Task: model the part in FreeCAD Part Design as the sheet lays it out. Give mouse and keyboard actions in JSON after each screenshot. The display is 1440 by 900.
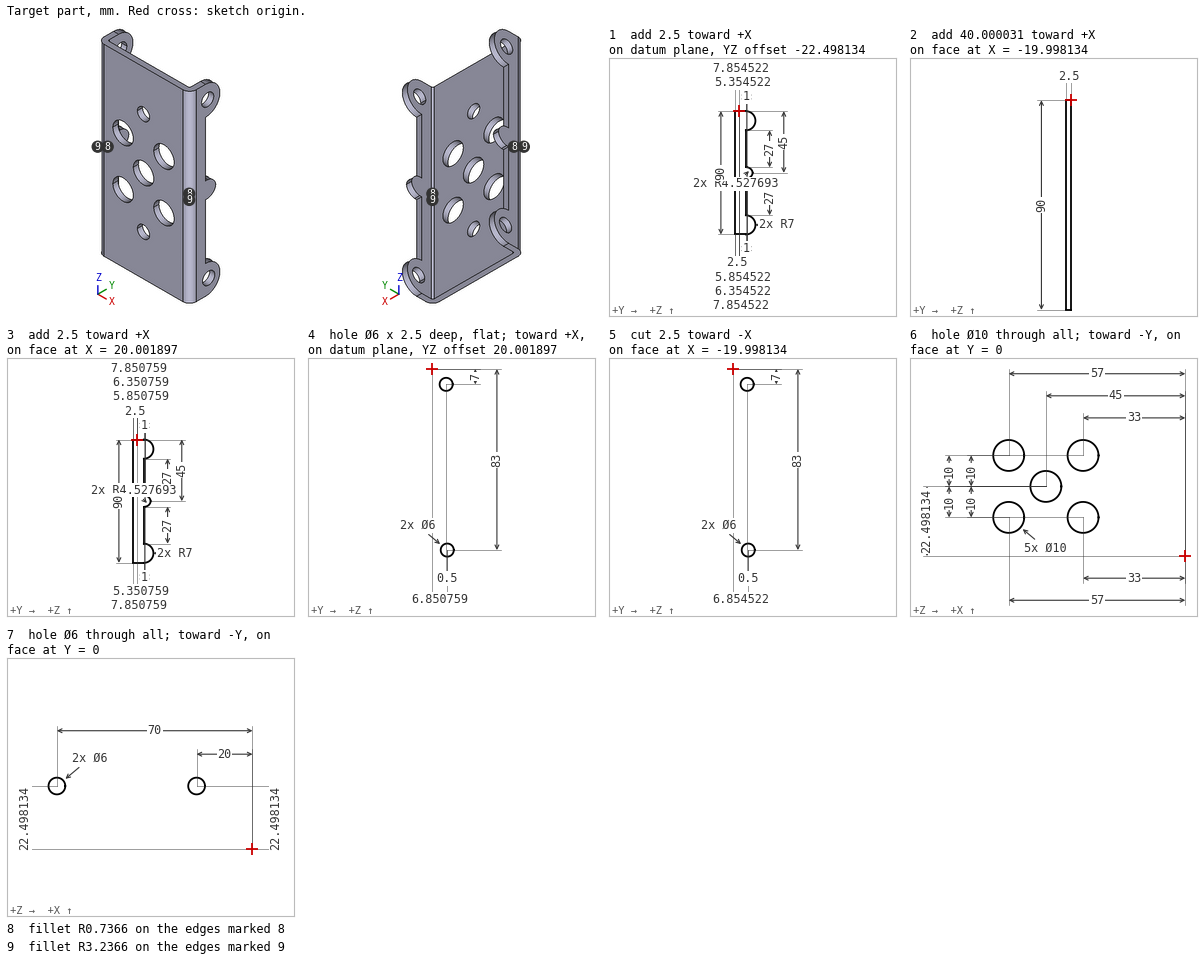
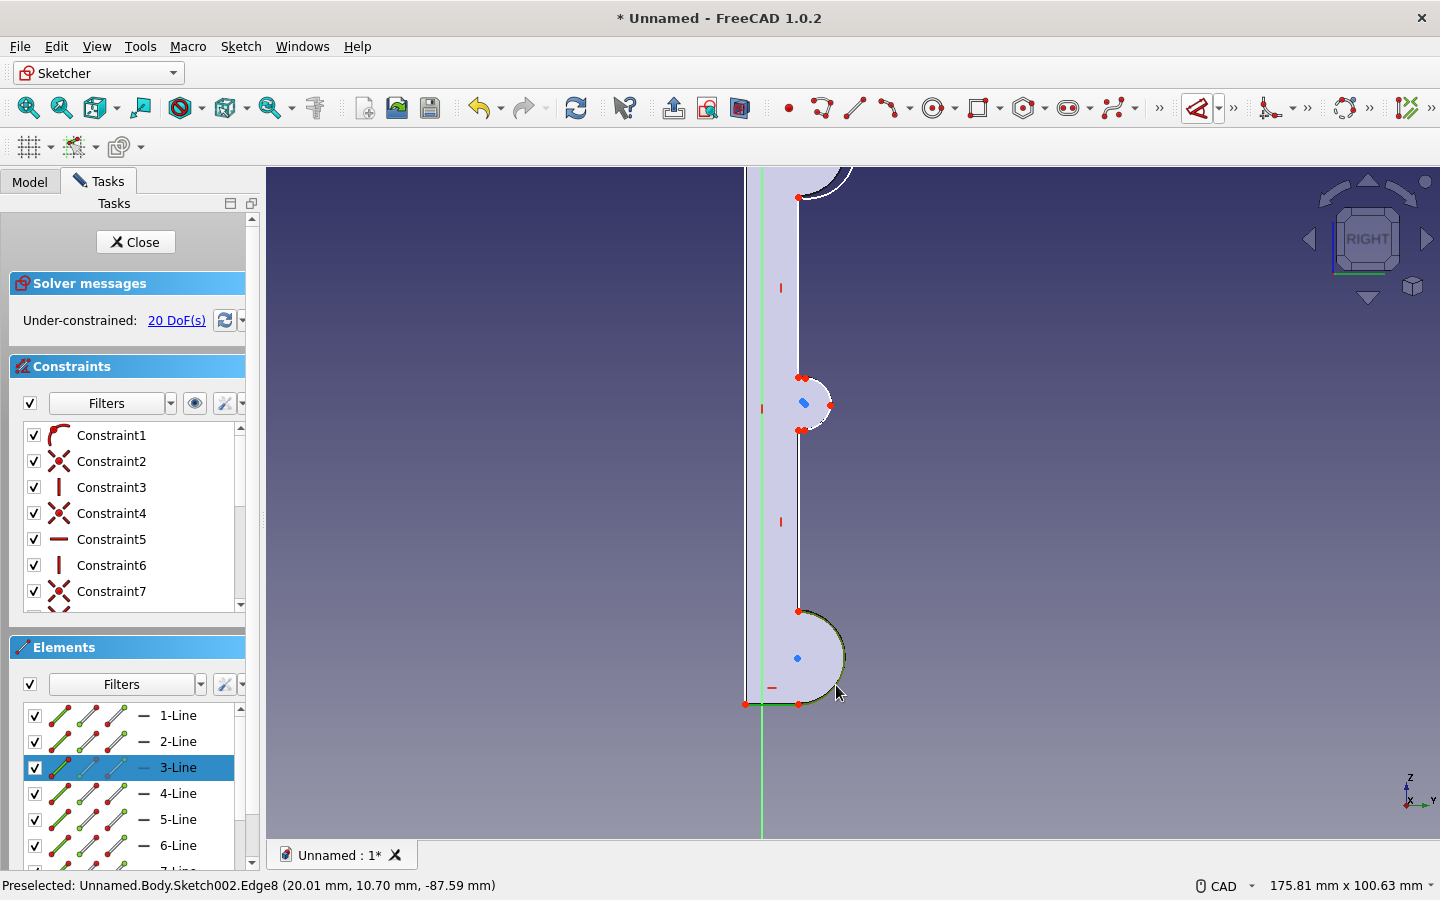
{"action": "key", "text": "t"}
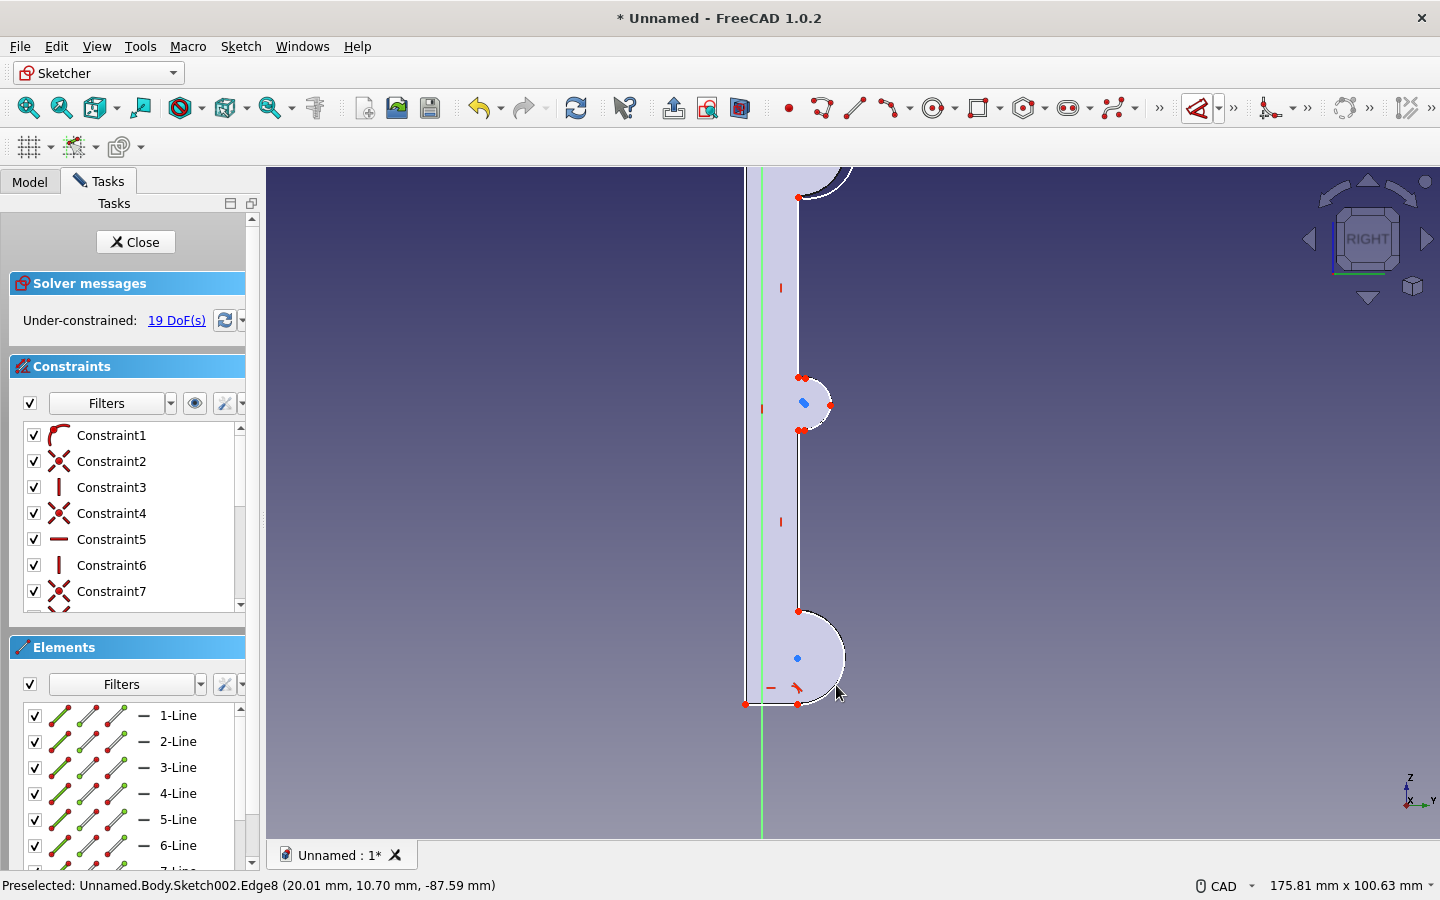
{"action": "scroll", "coordinate": [762, 706], "scroll_direction": "down", "scroll_amount": 2}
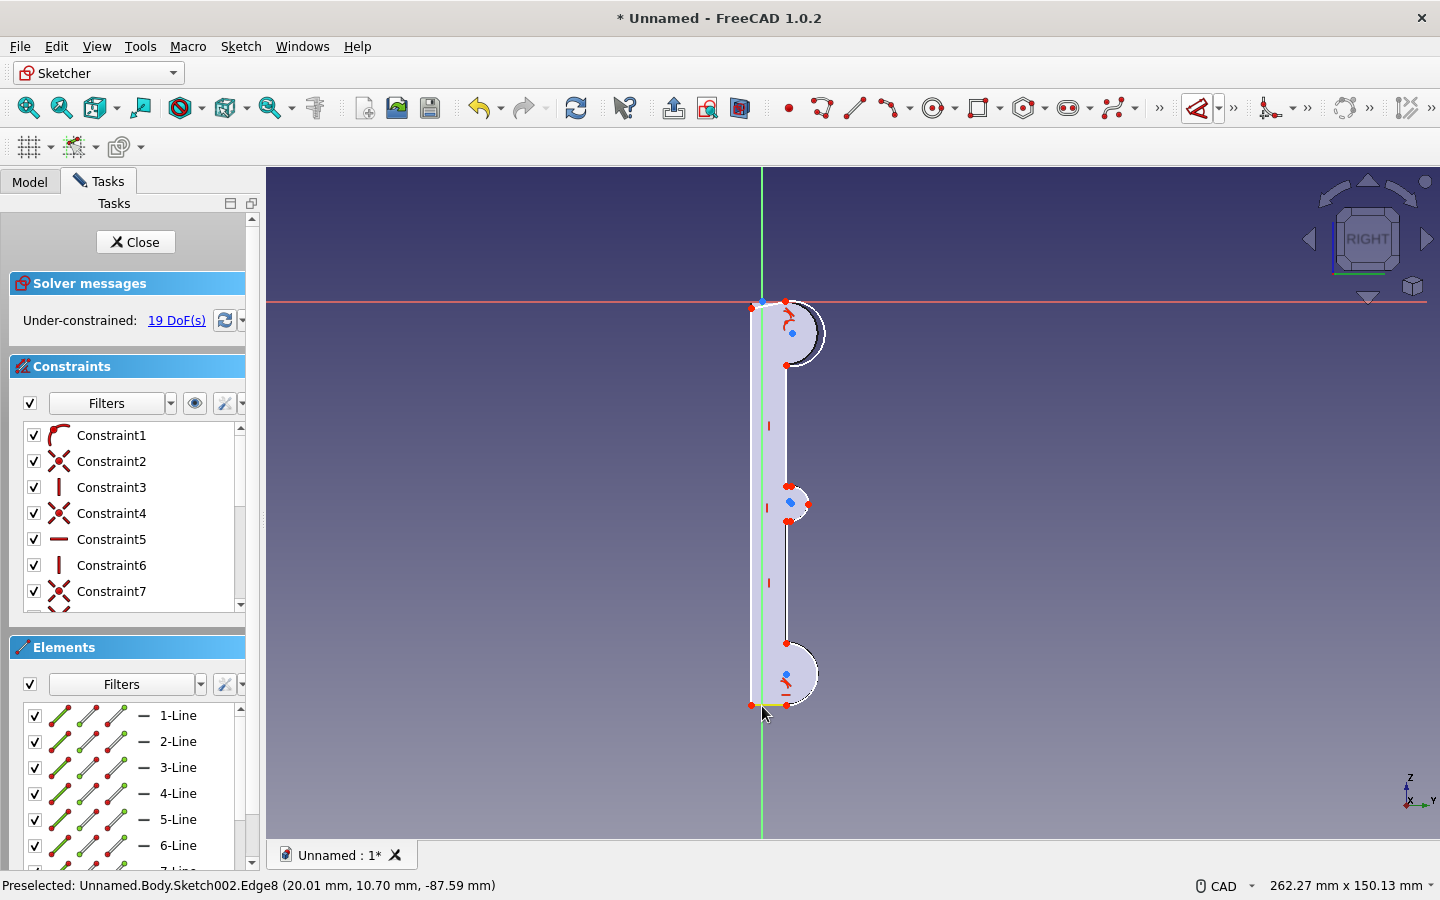
{"action": "scroll", "coordinate": [775, 304], "scroll_direction": "up", "scroll_amount": 2}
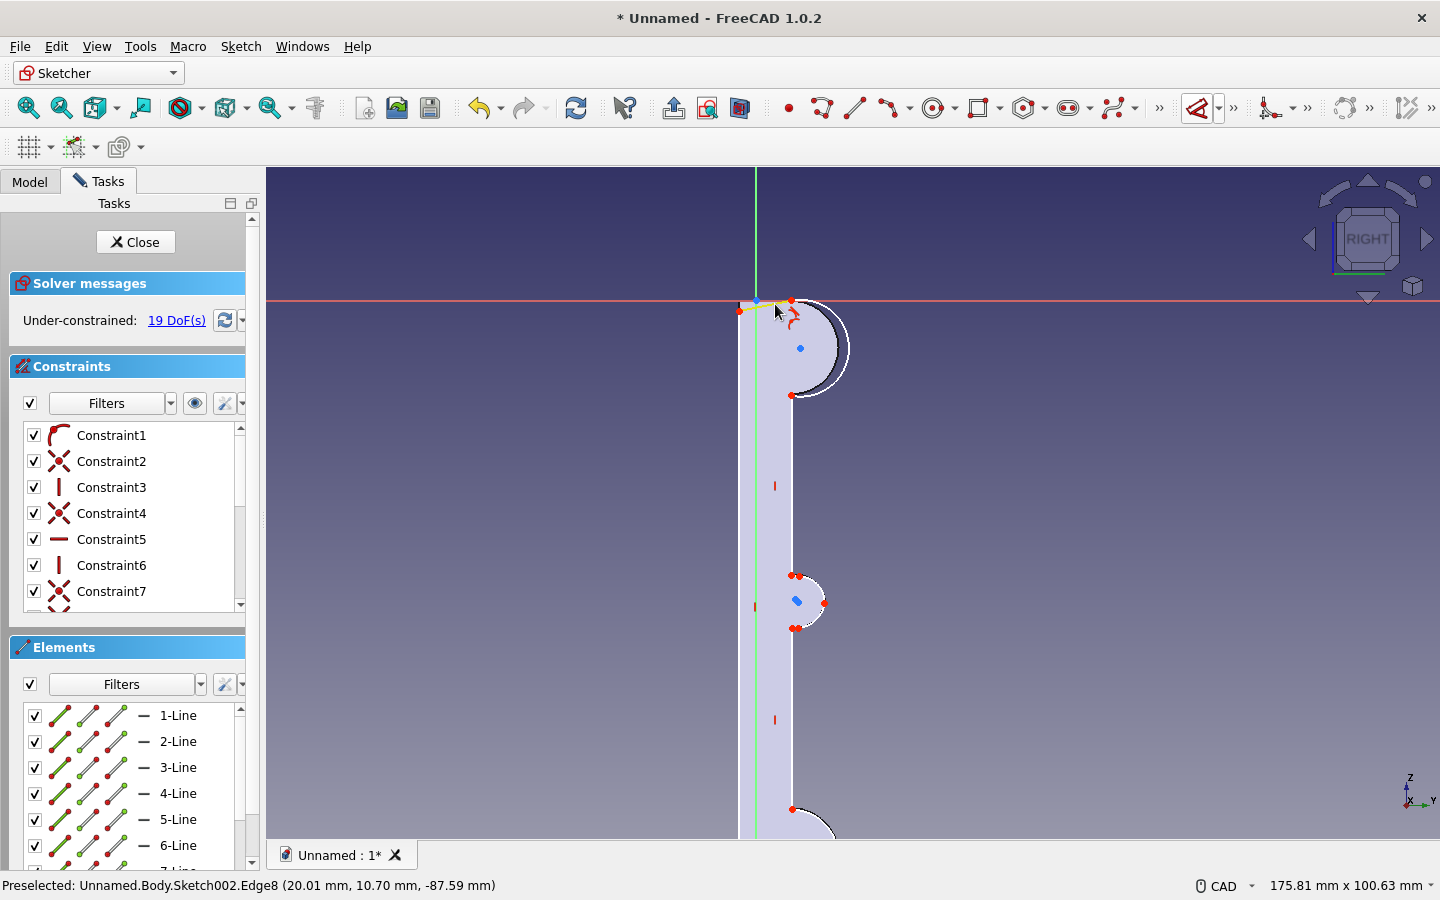
{"action": "left_click", "coordinate": [775, 304]}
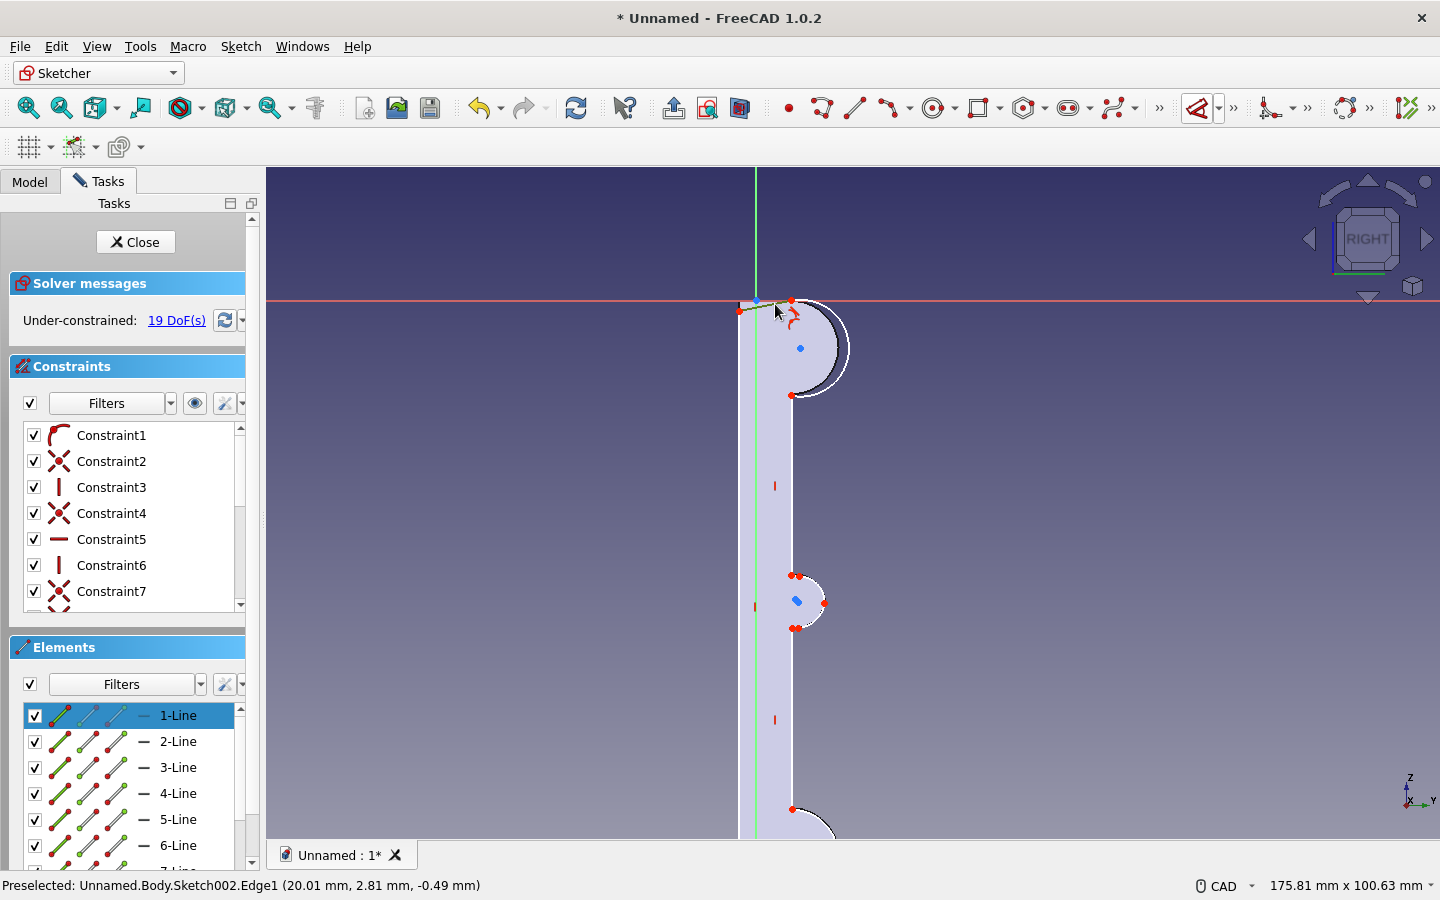
{"action": "key", "text": "h"}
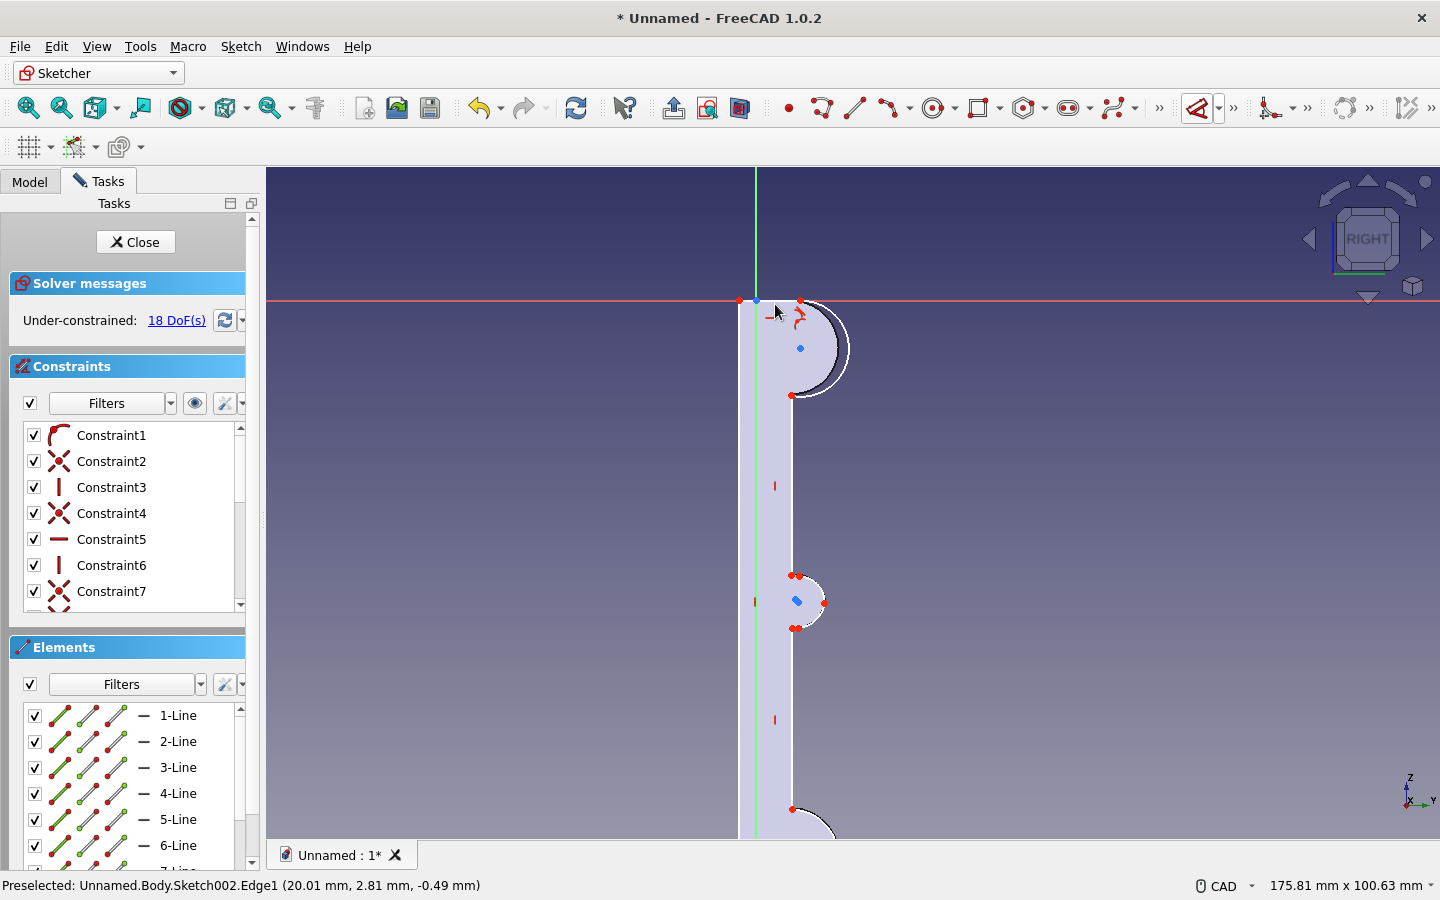
{"action": "scroll", "coordinate": [795, 628], "scroll_direction": "up", "scroll_amount": 8}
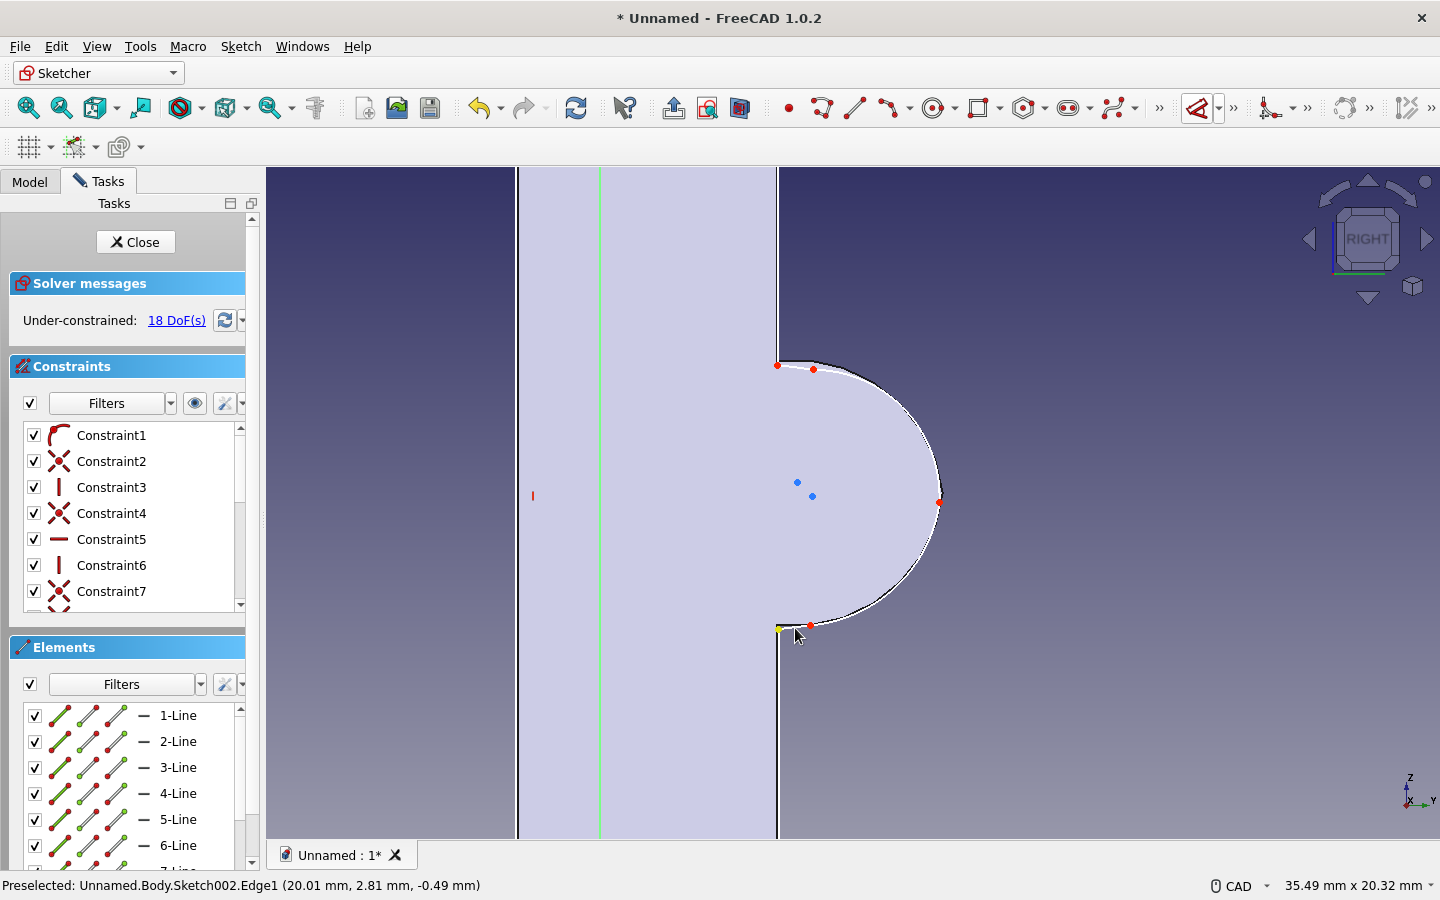
{"action": "left_click", "coordinate": [795, 627]}